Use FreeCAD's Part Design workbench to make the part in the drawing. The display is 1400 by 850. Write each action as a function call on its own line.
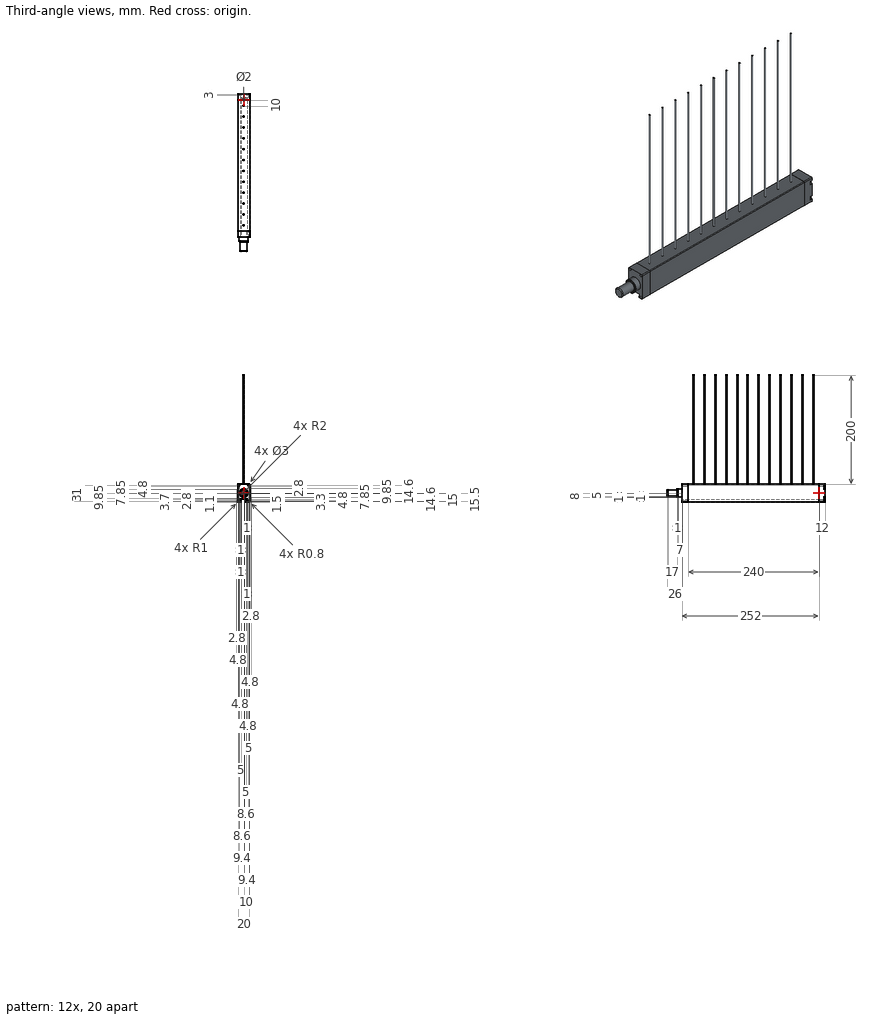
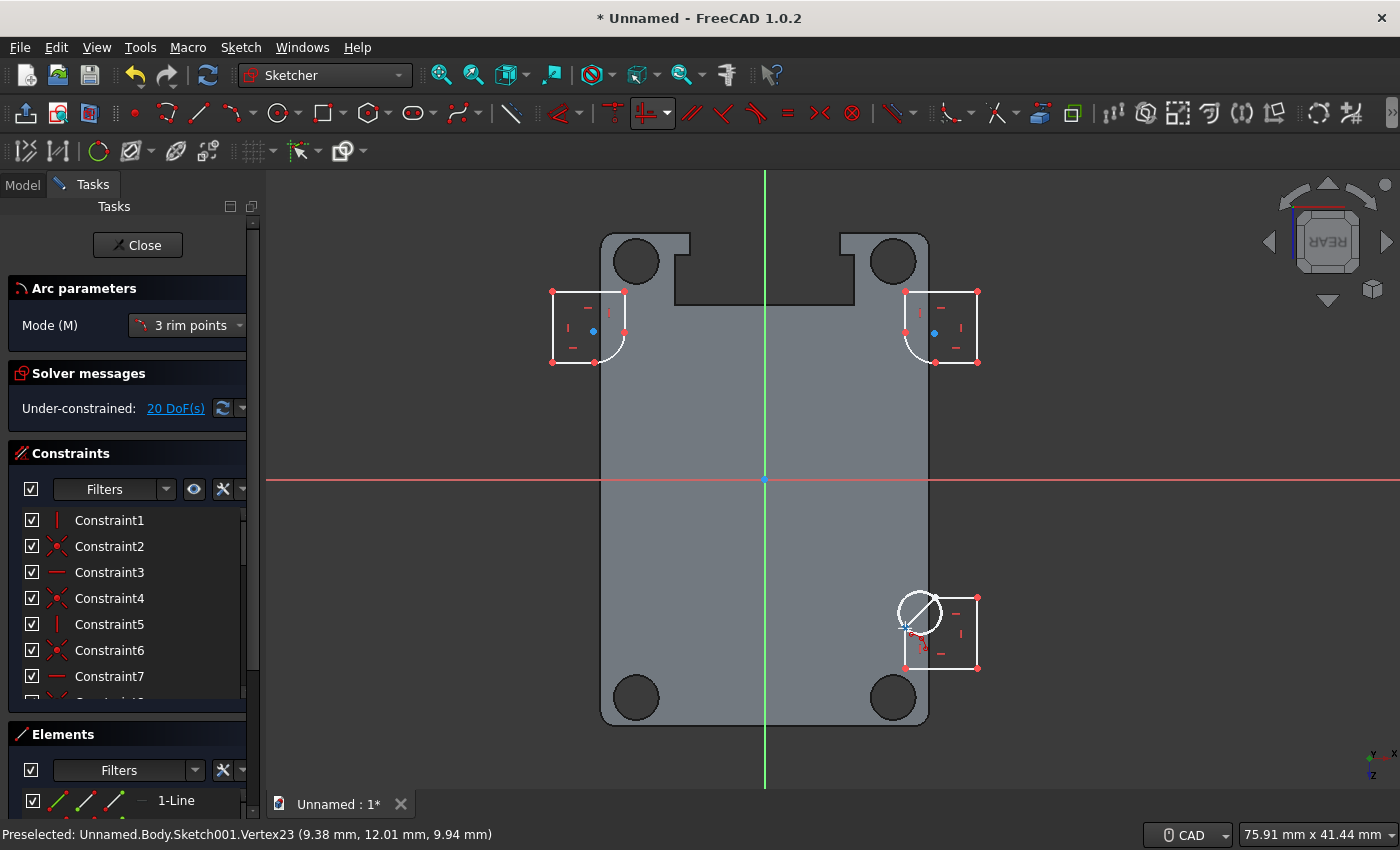
scroll(914, 606, up, 3)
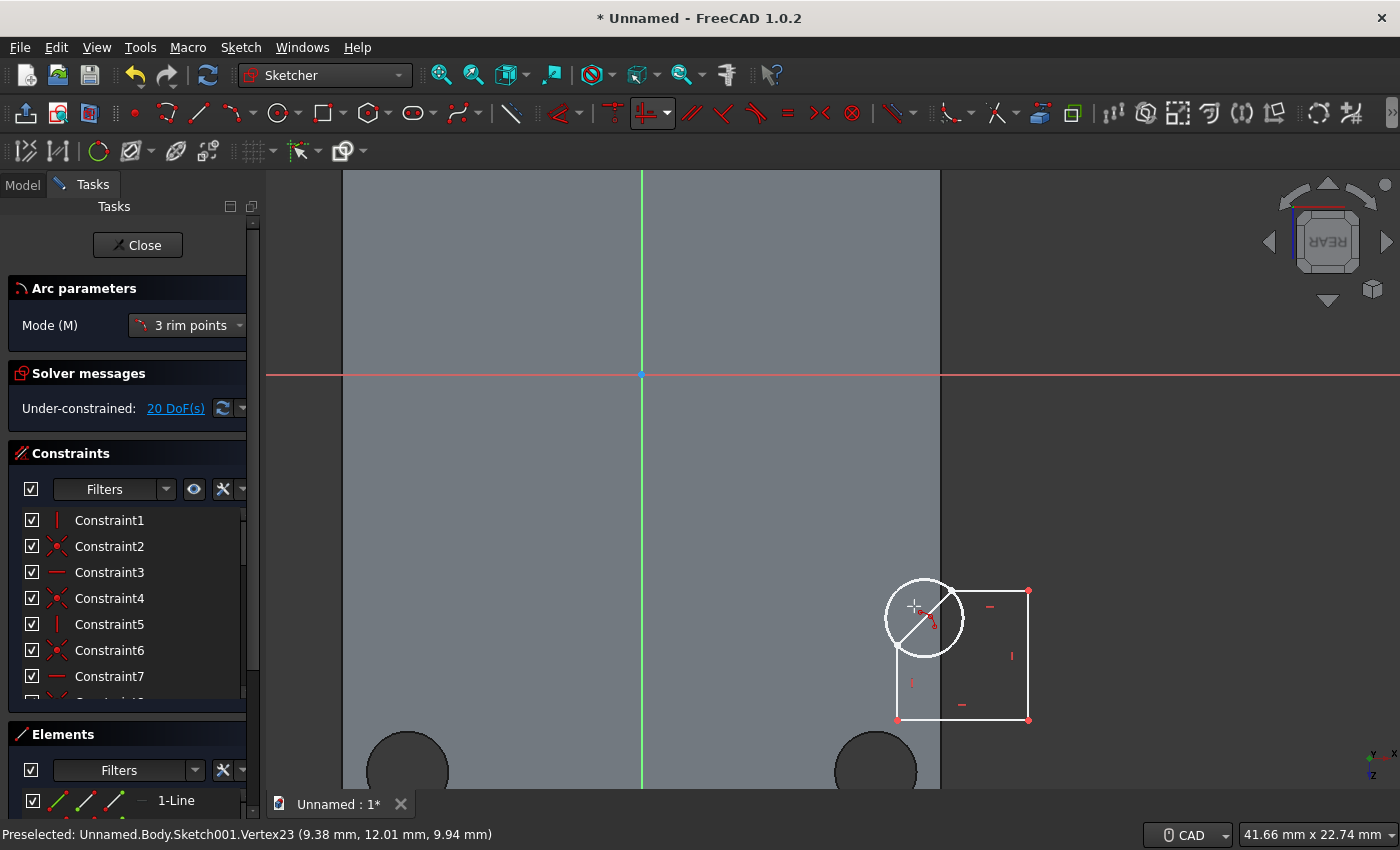
click(913, 605)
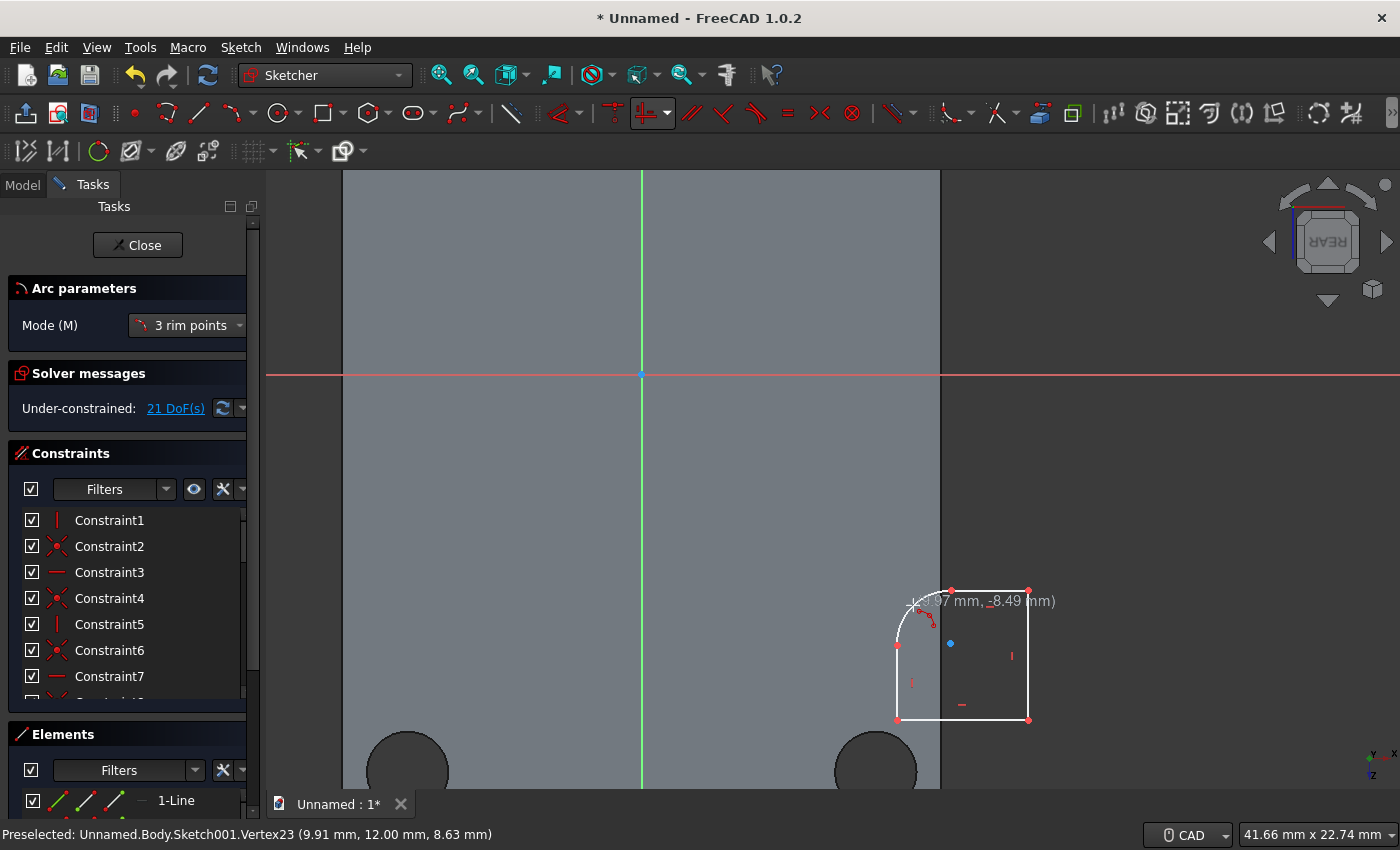
click(168, 114)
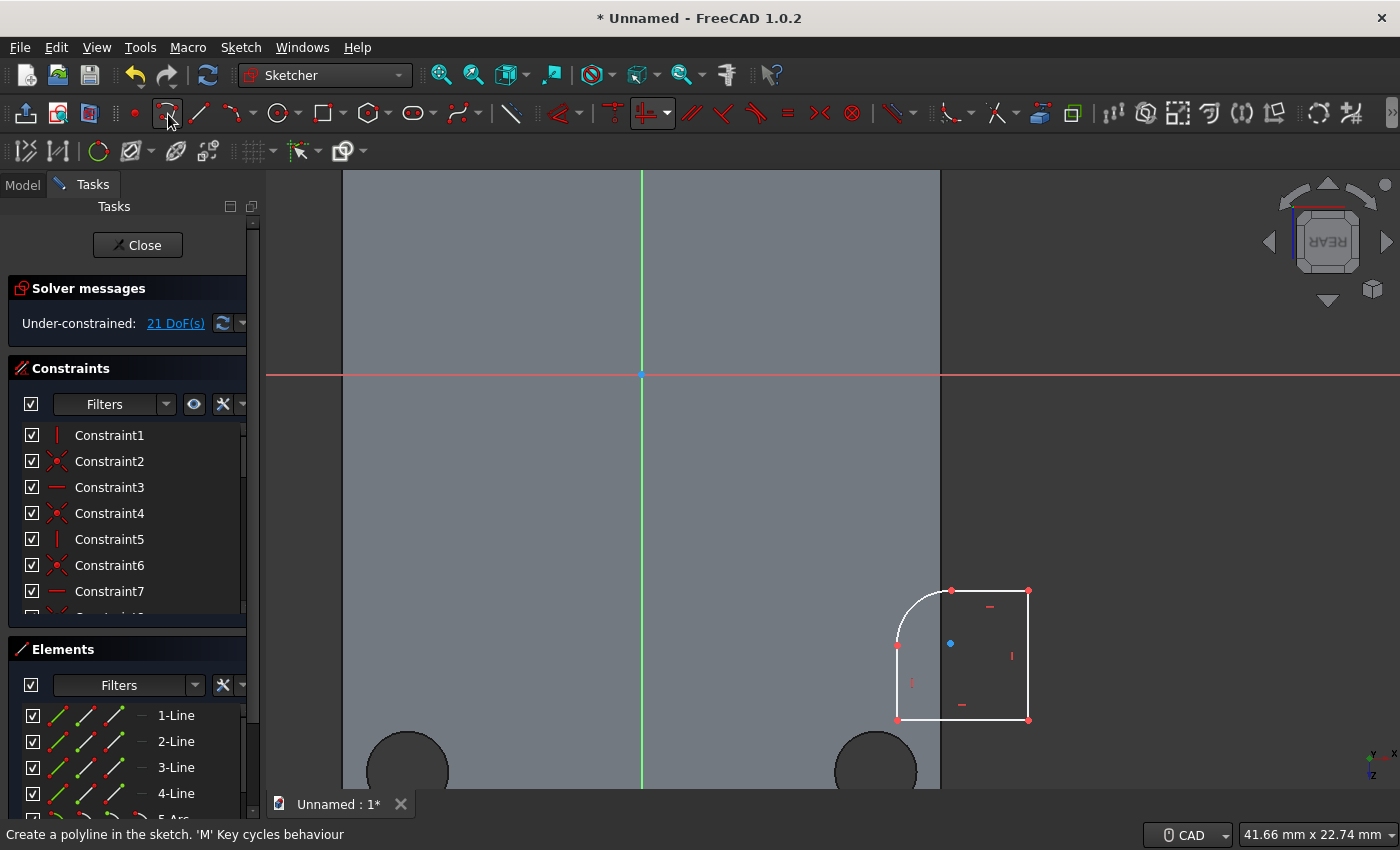
click(331, 589)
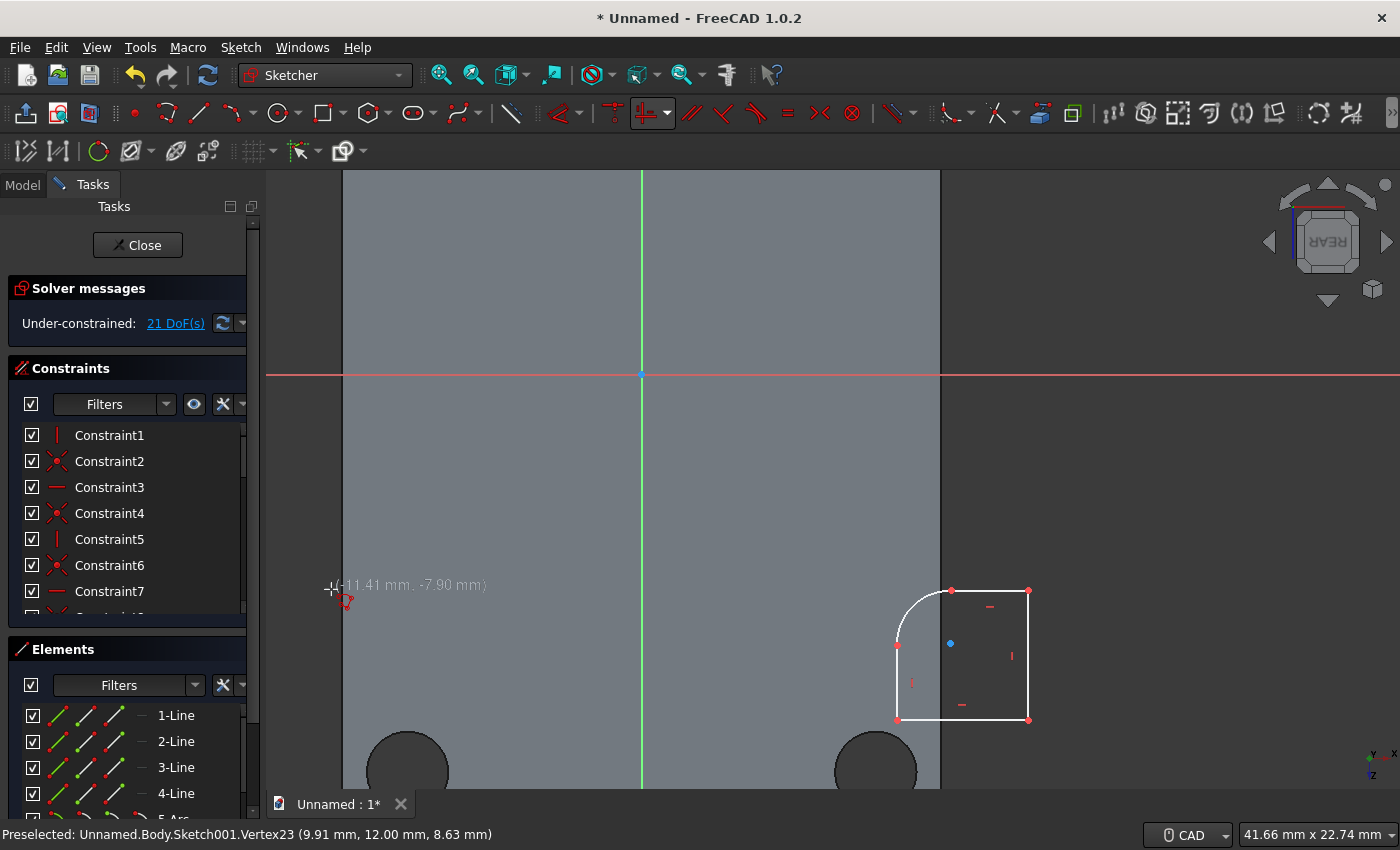
scroll(914, 607, down, 3)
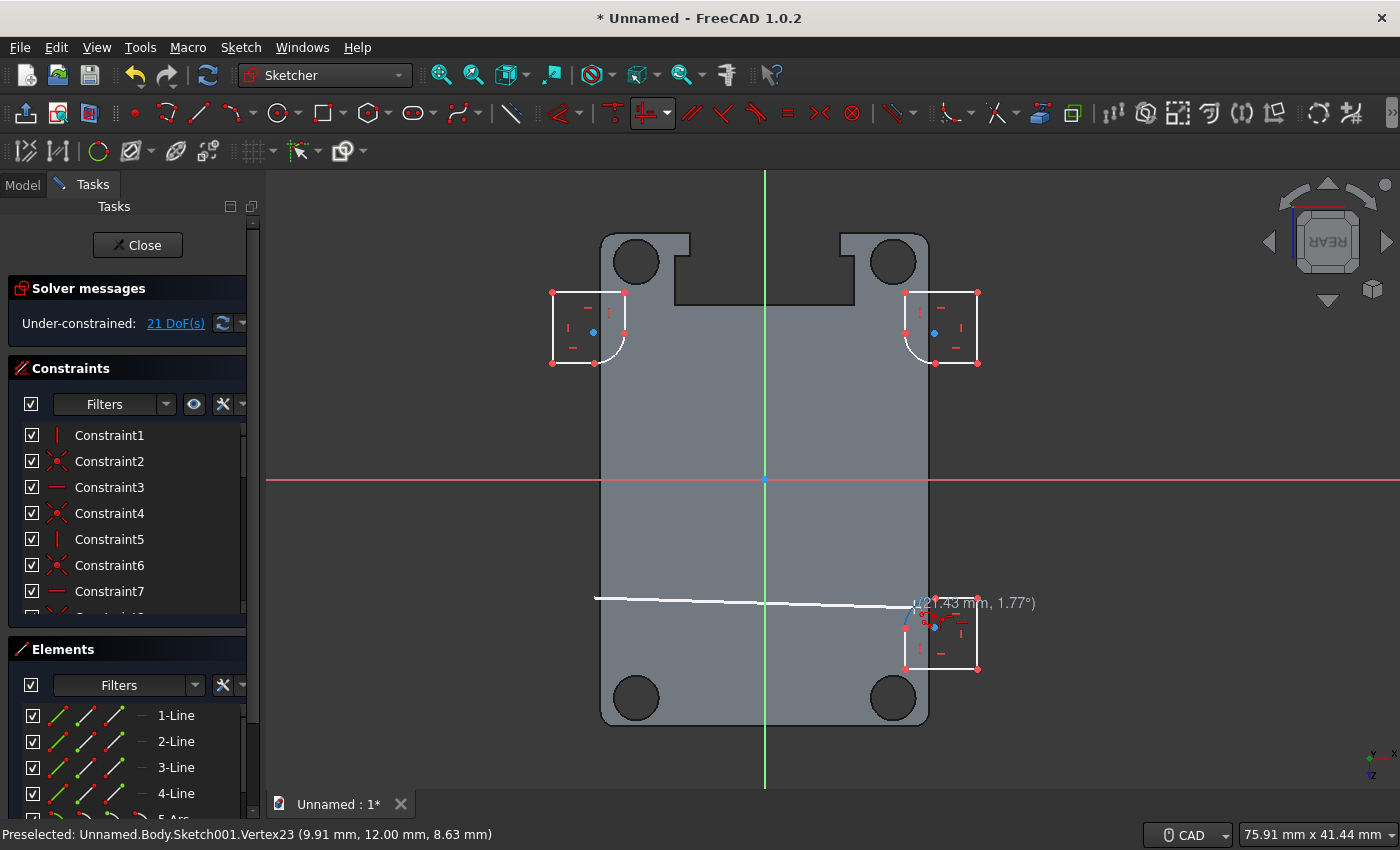
click(553, 597)
click(553, 669)
click(624, 669)
click(624, 627)
right_click(624, 627)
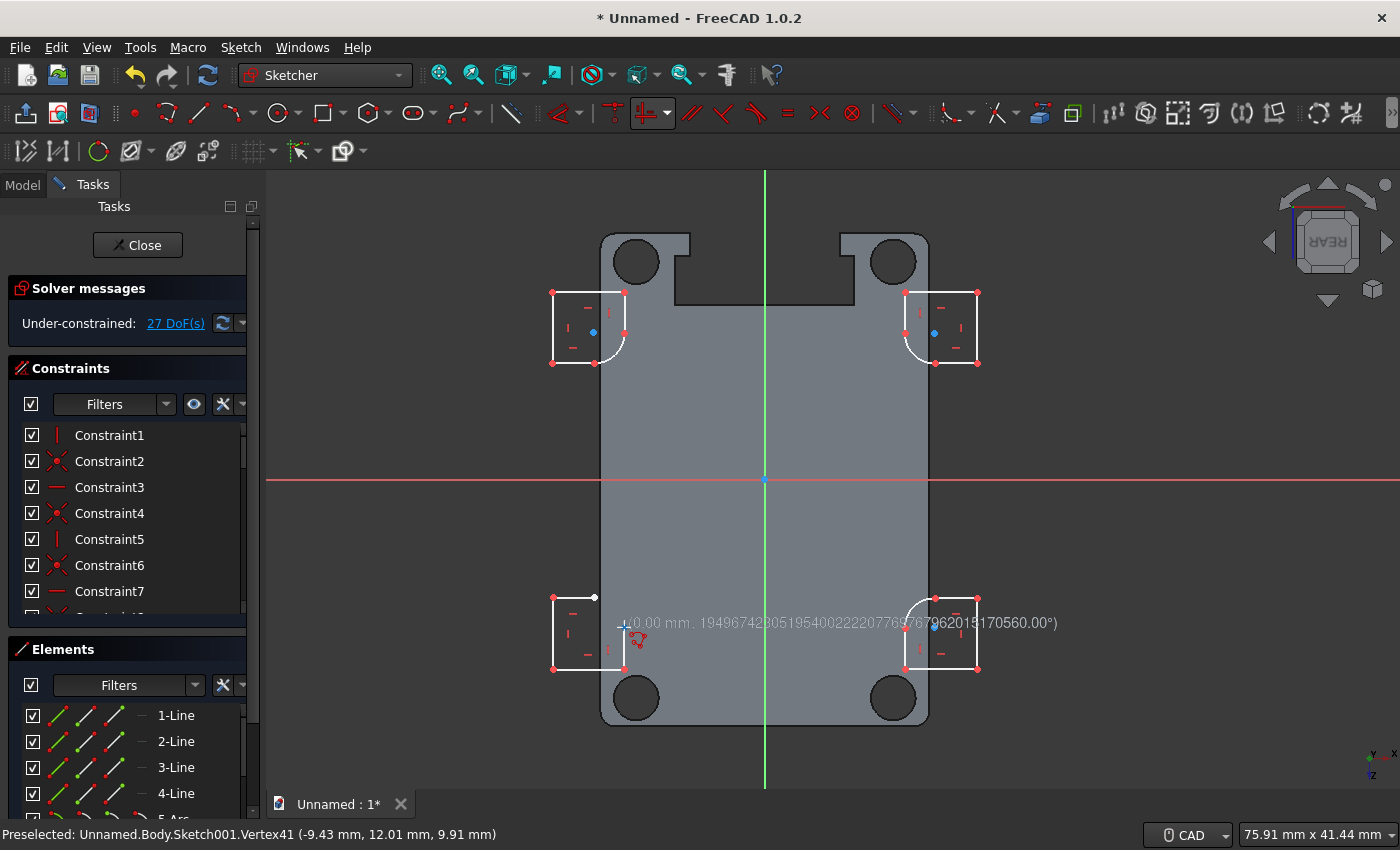
click(232, 114)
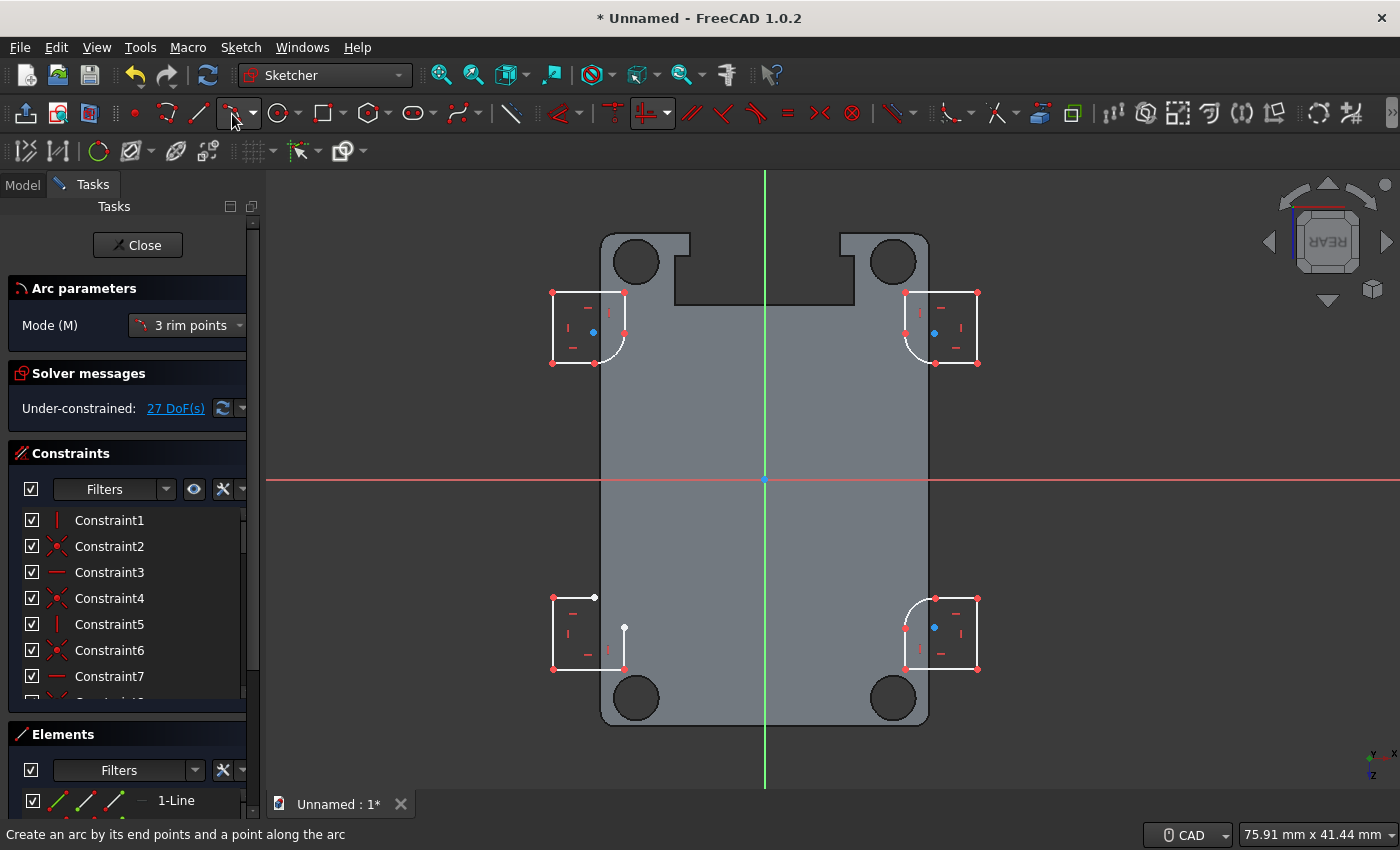
click(624, 628)
click(594, 598)